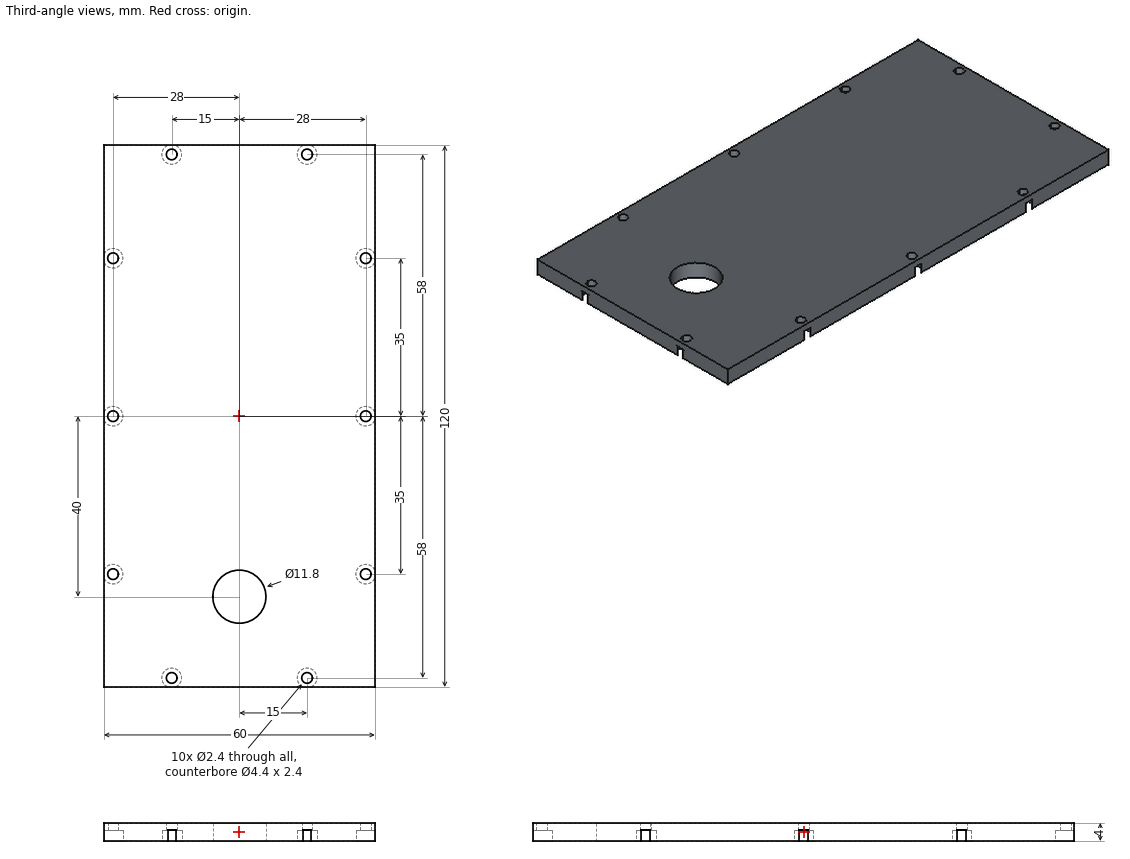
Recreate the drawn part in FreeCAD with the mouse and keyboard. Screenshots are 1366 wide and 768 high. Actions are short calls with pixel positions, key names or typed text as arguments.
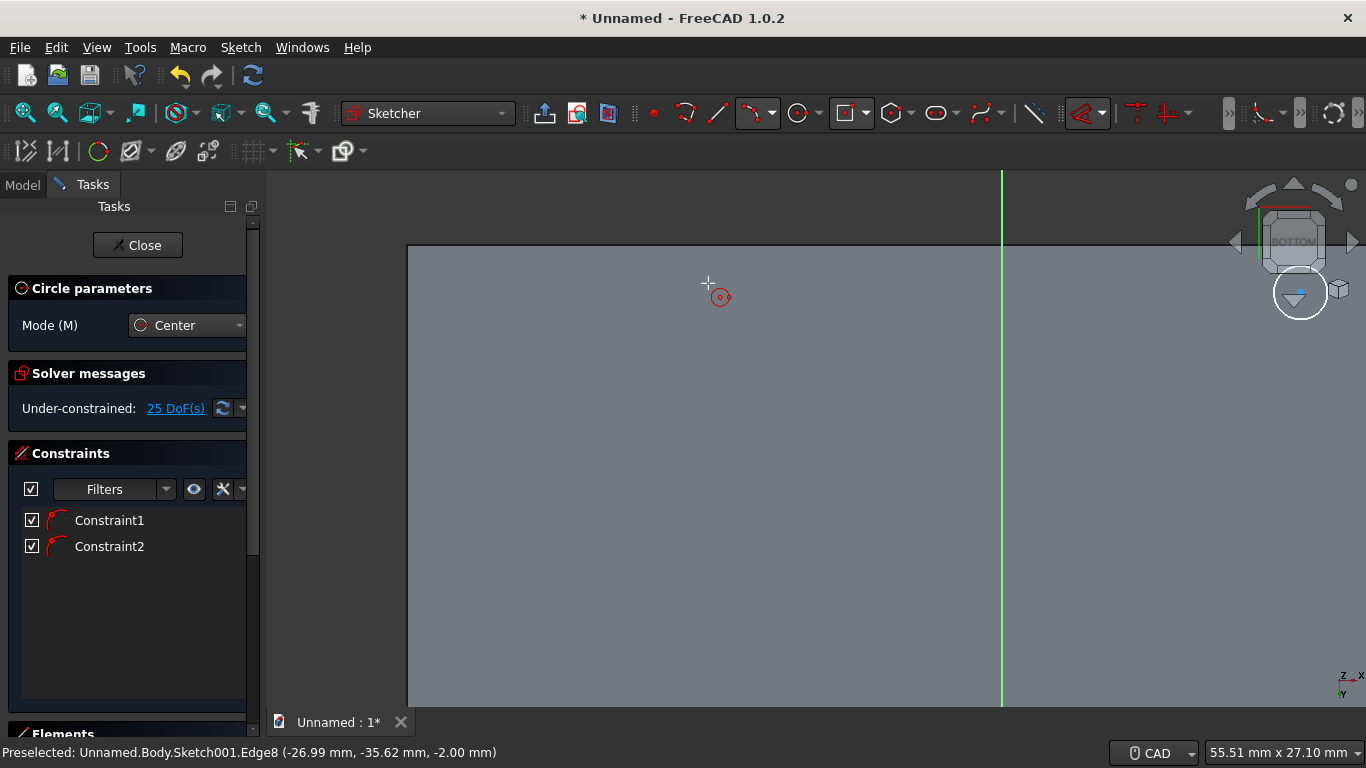
scroll(708, 283, down, 10)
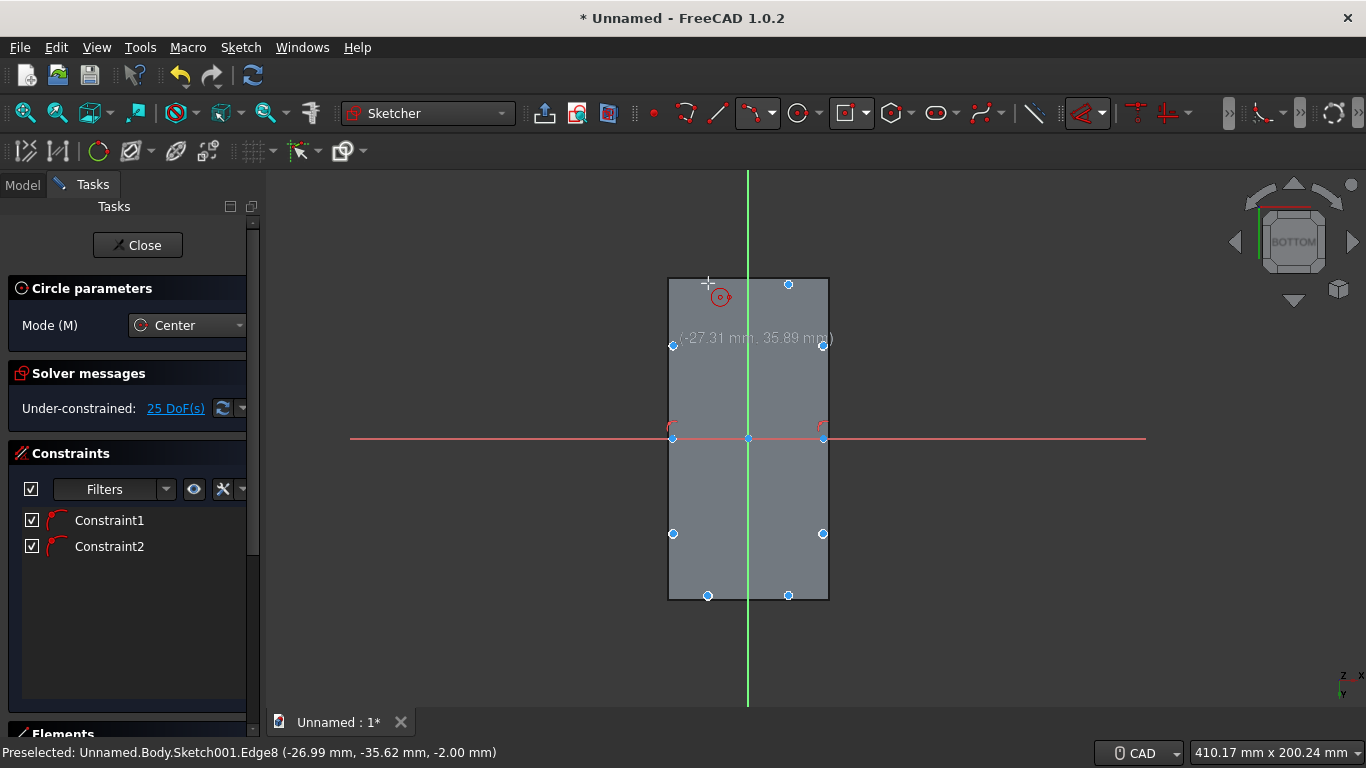
click(708, 283)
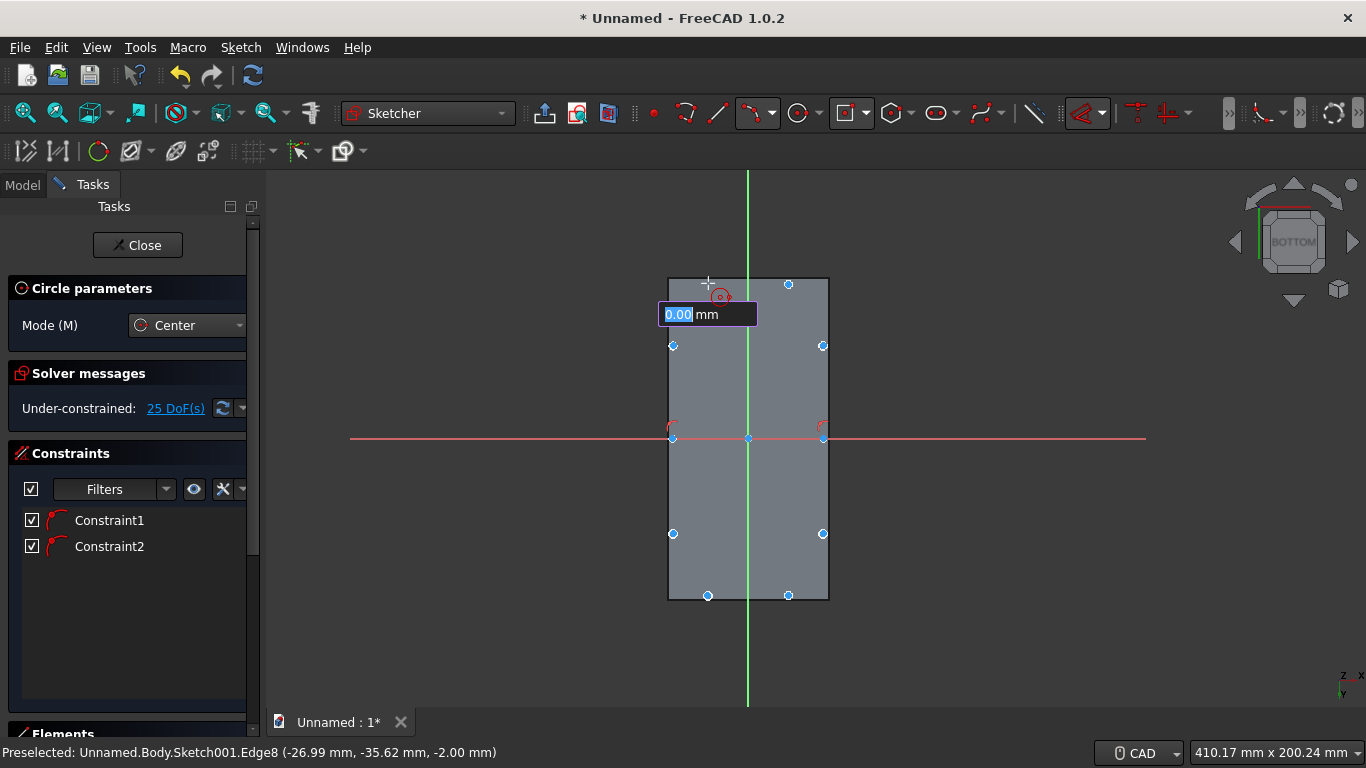
scroll(710, 281, up, 8)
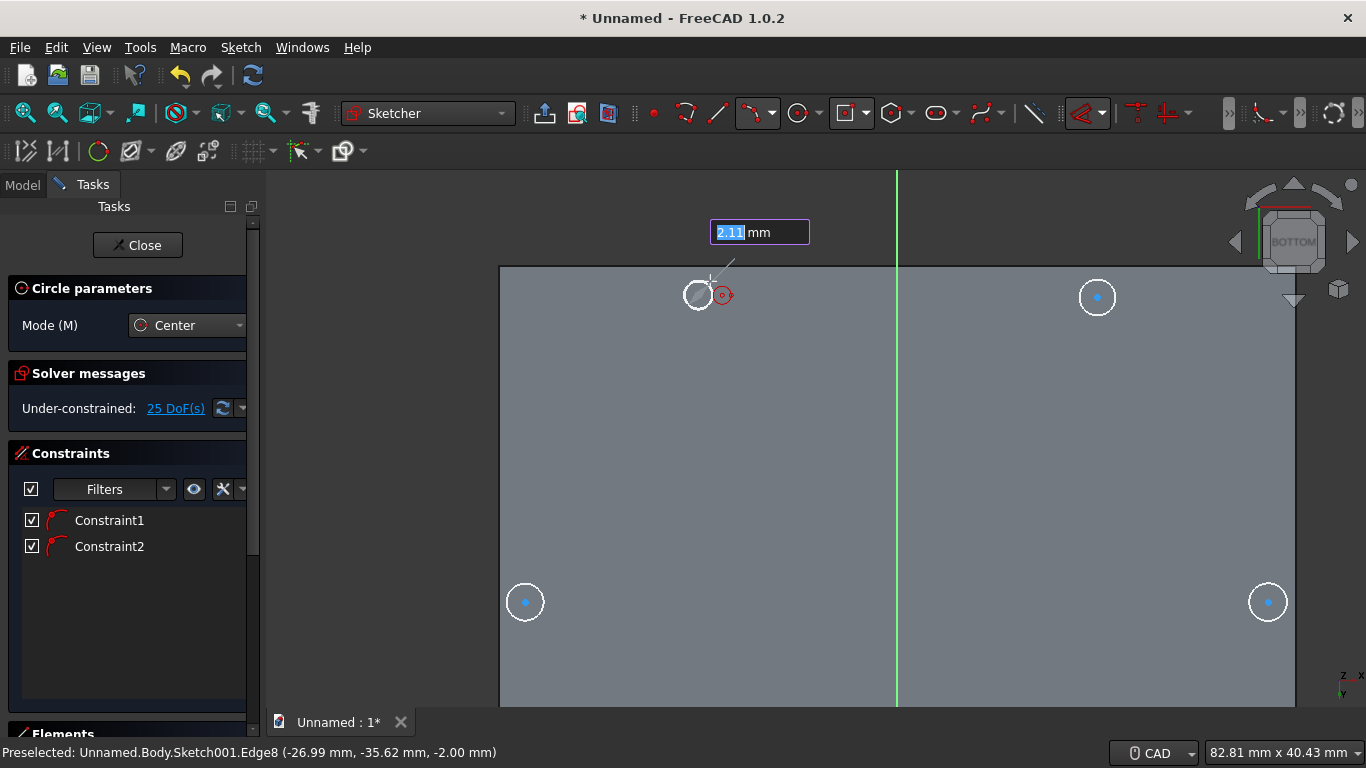
click(709, 281)
key(Escape)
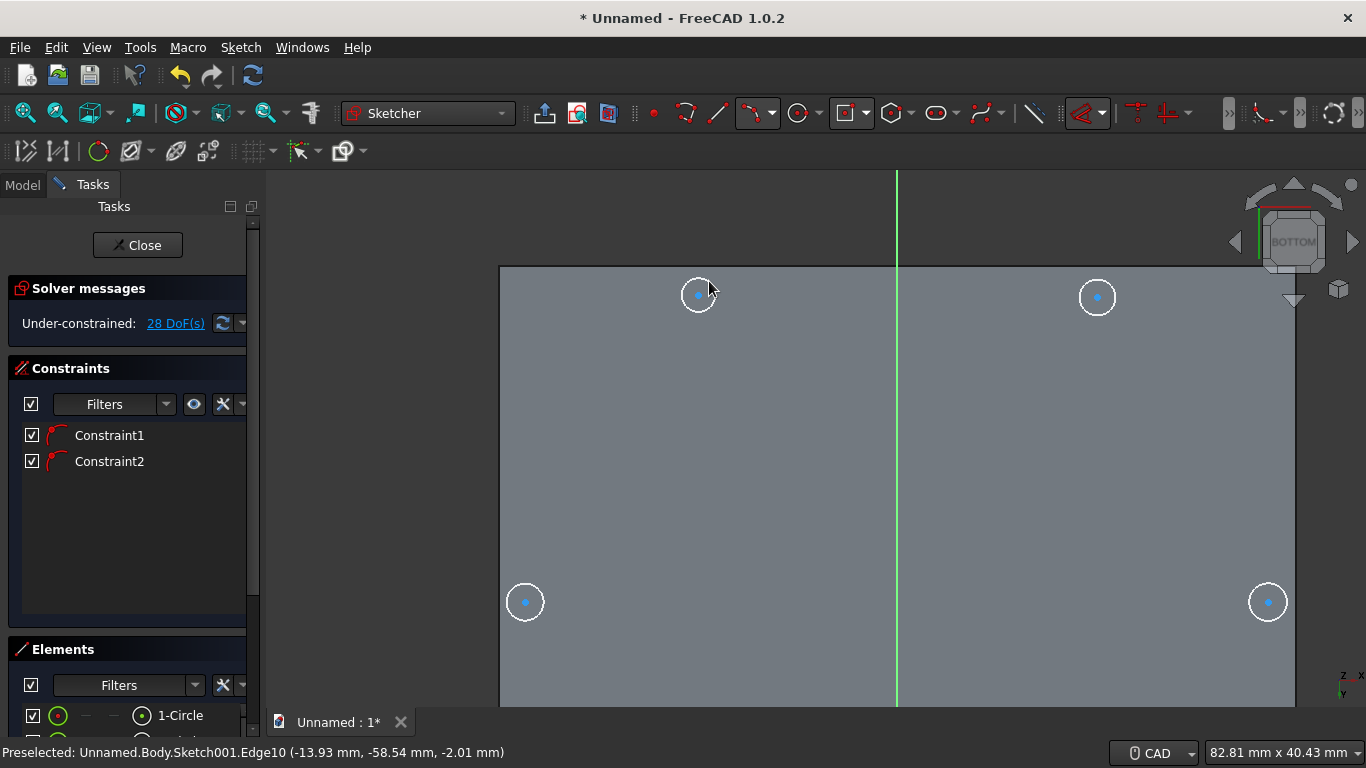
click(1110, 285)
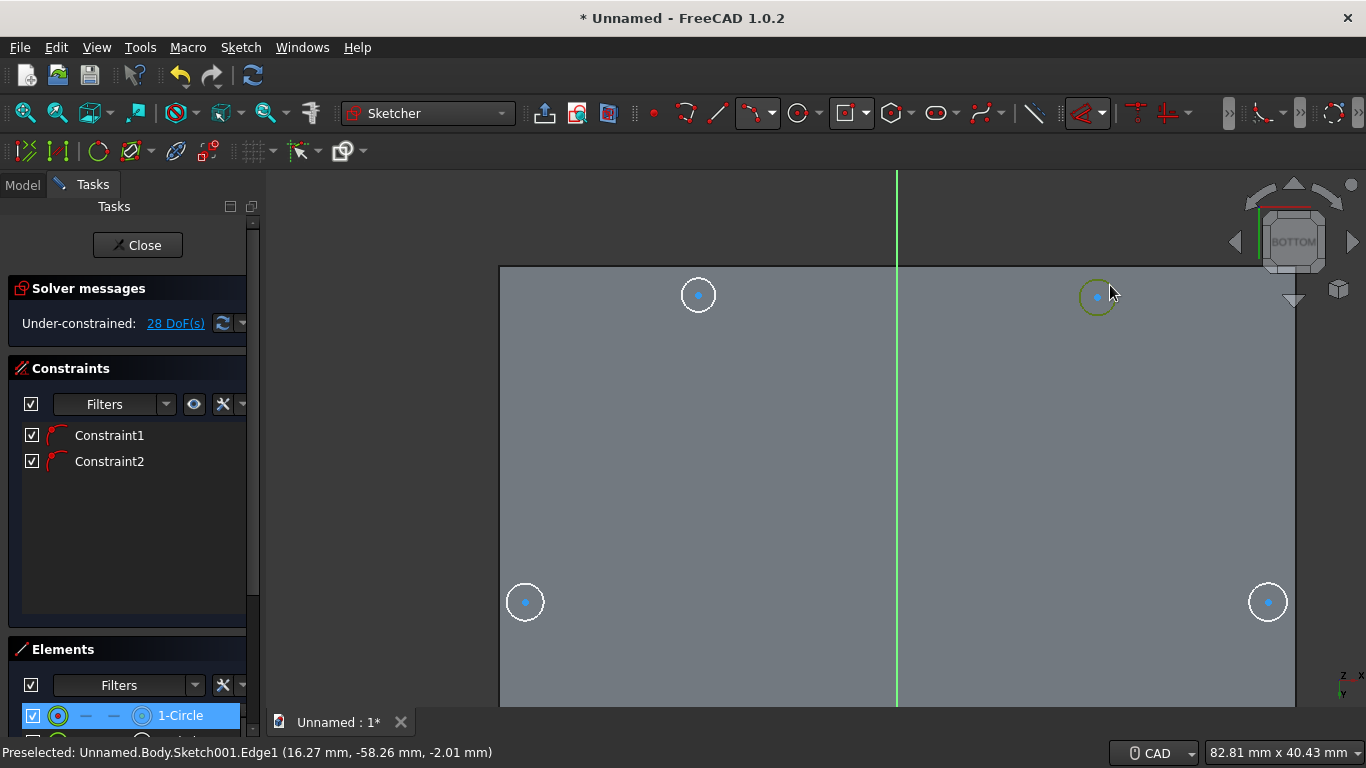
scroll(710, 281, down, 8)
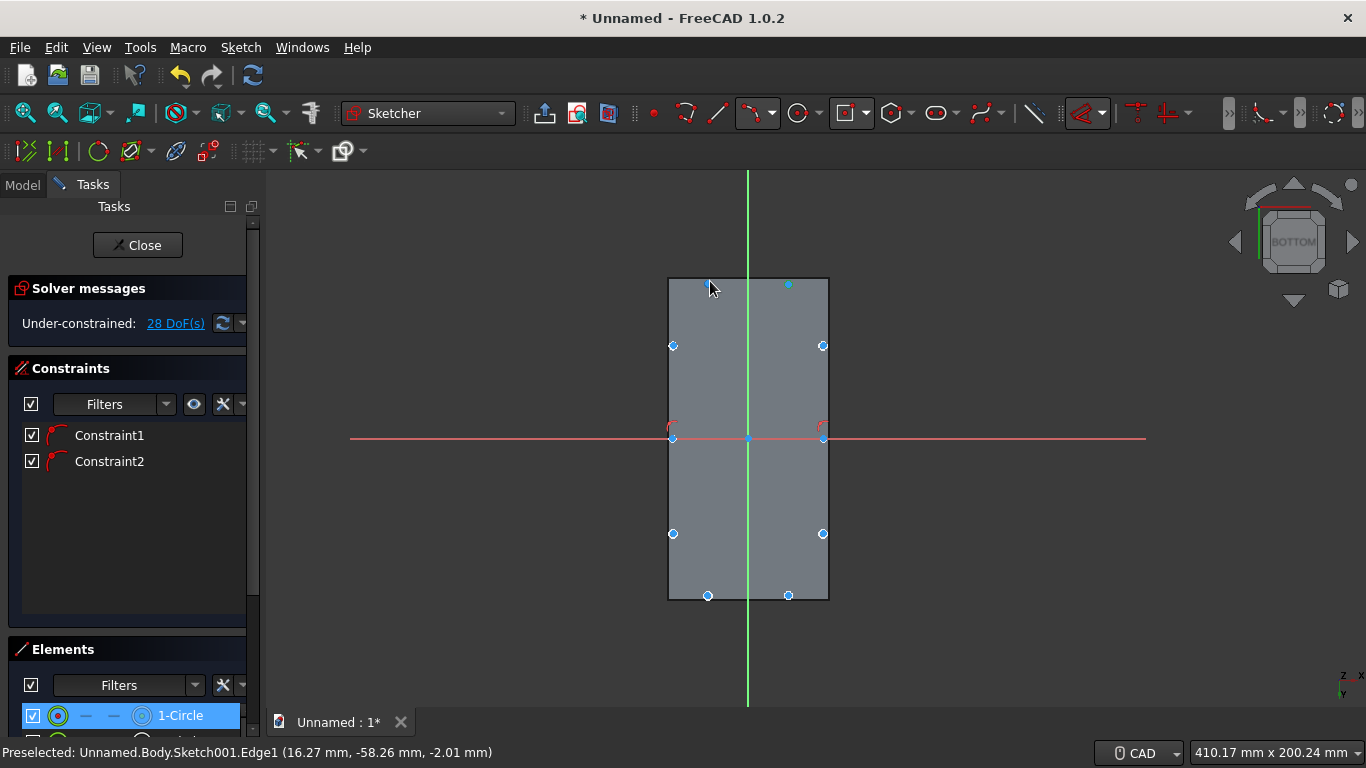
scroll(826, 437, up, 10)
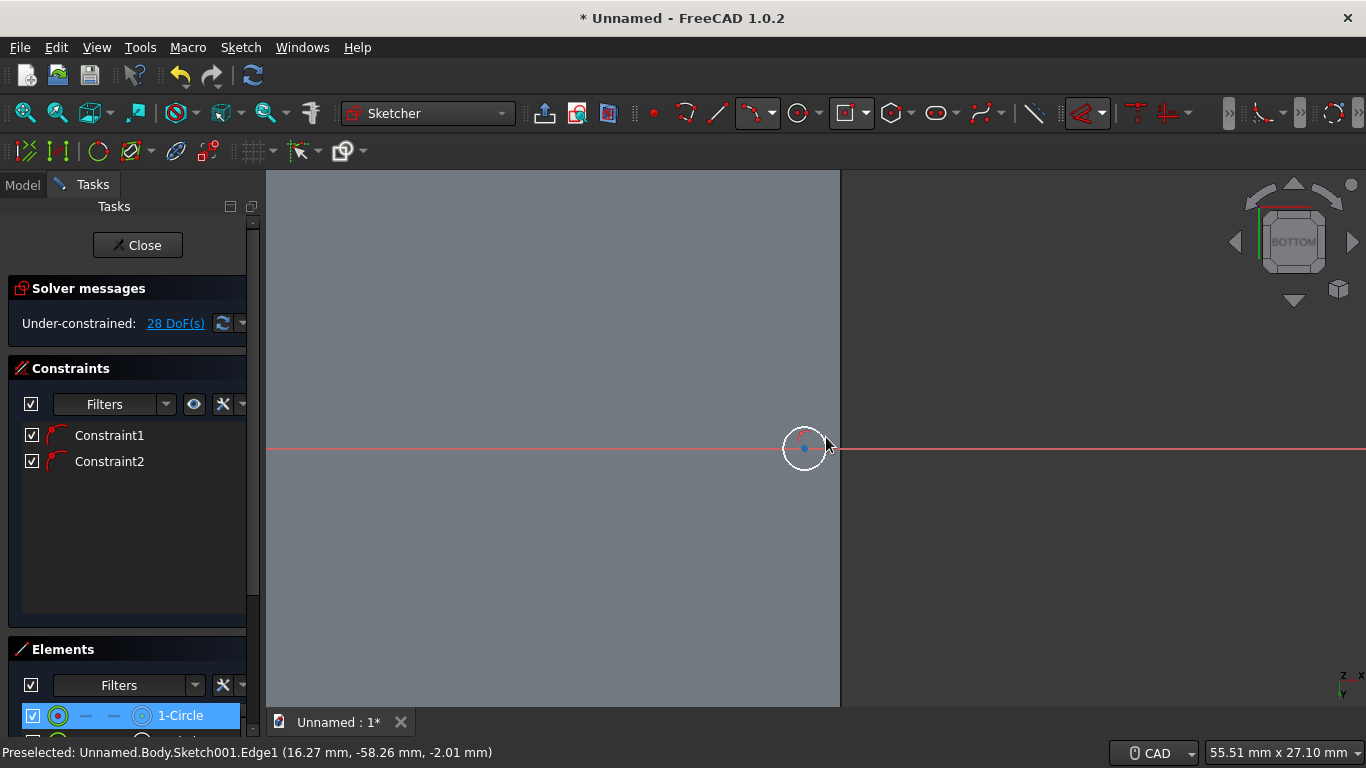
click(820, 433)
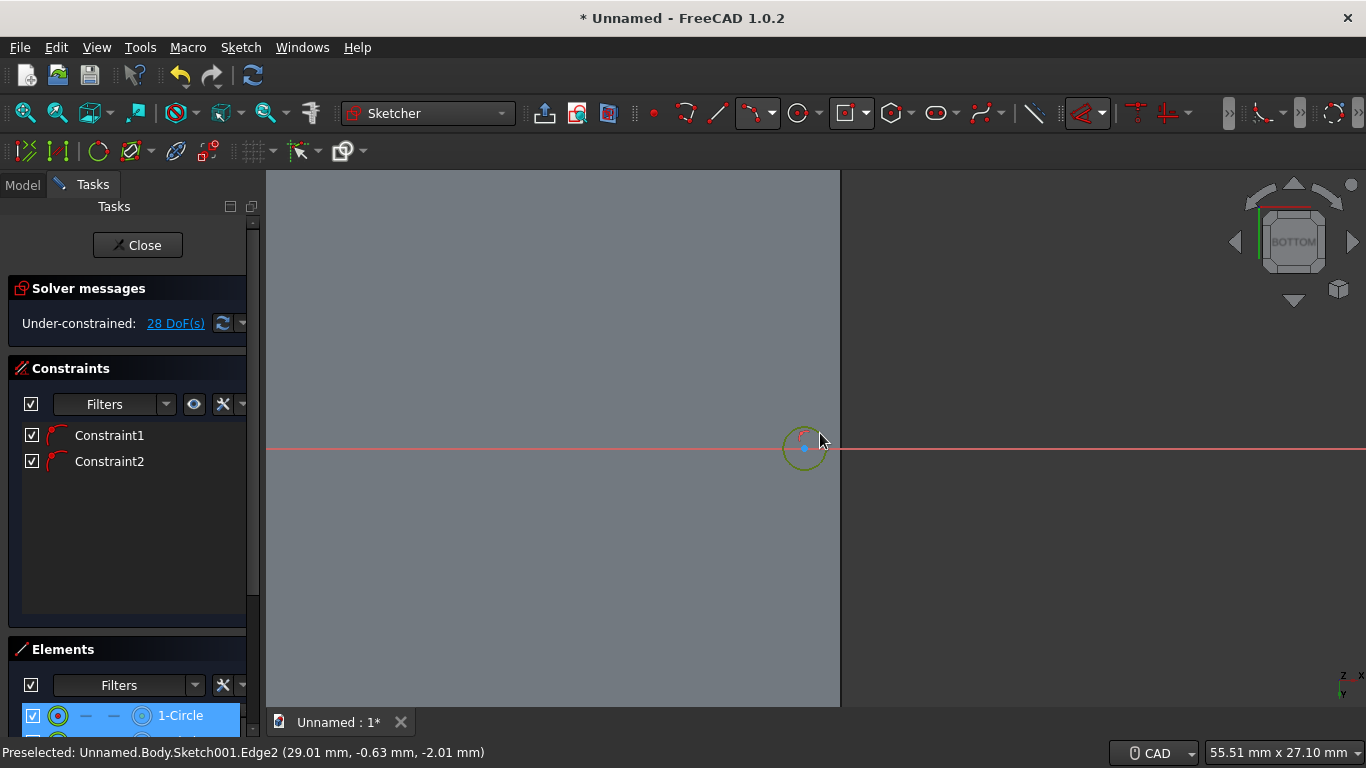
scroll(826, 437, down, 10)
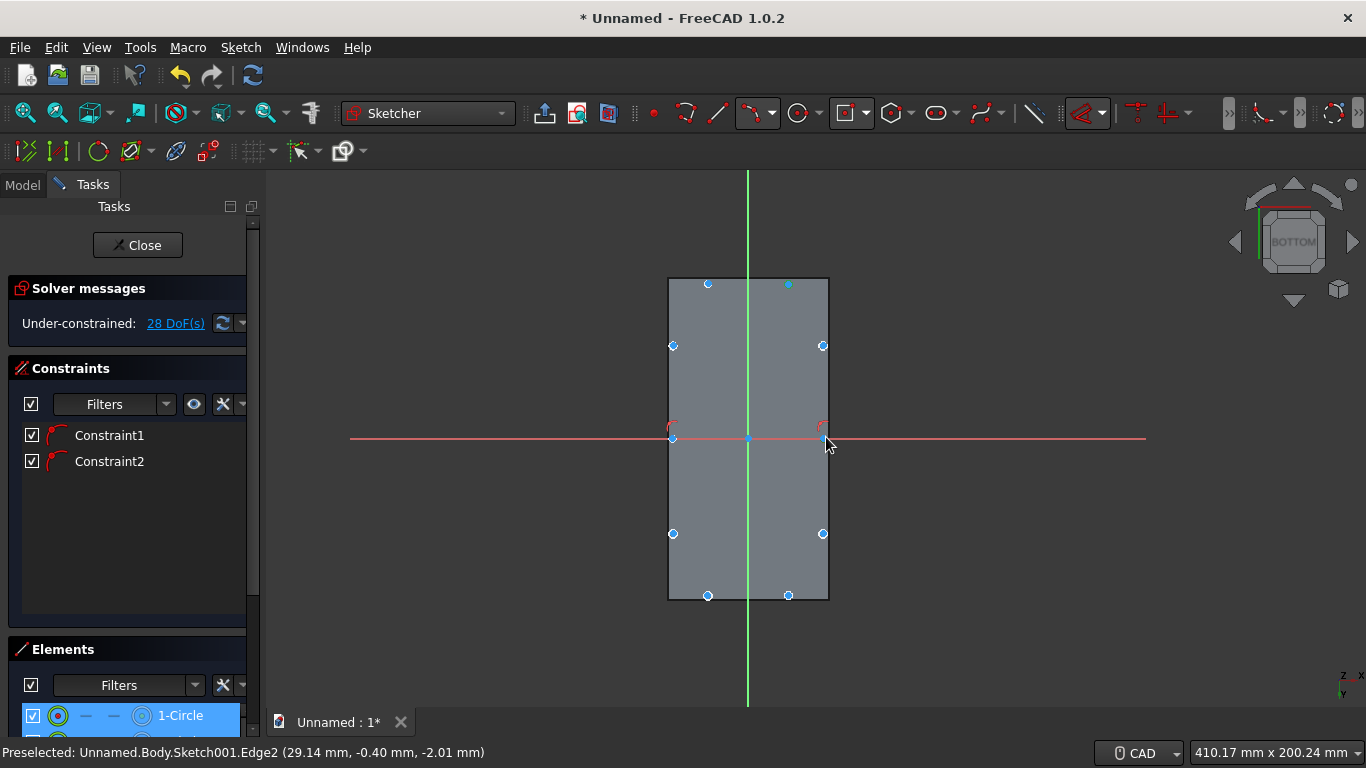
scroll(675, 437, up, 10)